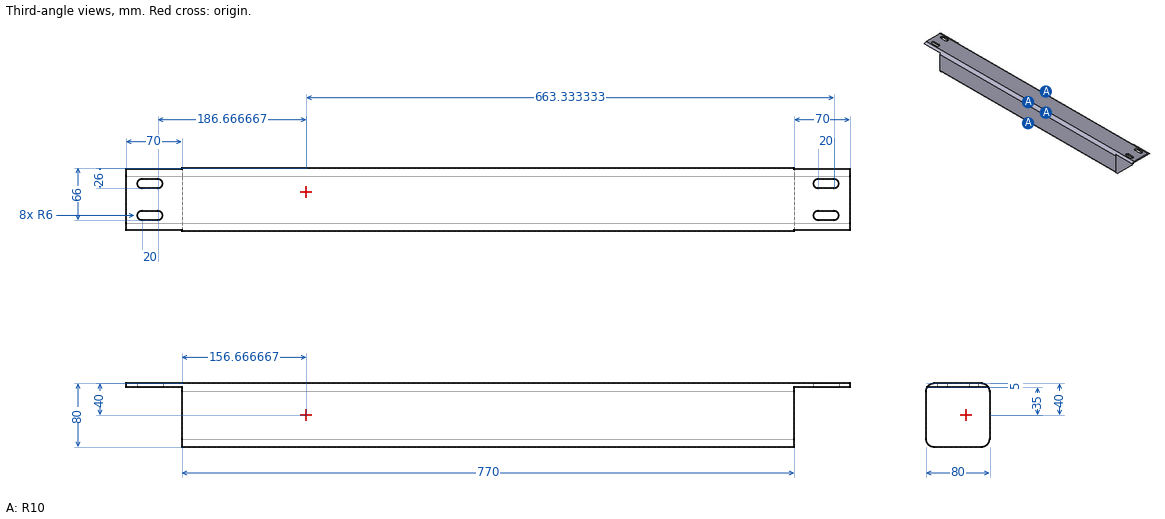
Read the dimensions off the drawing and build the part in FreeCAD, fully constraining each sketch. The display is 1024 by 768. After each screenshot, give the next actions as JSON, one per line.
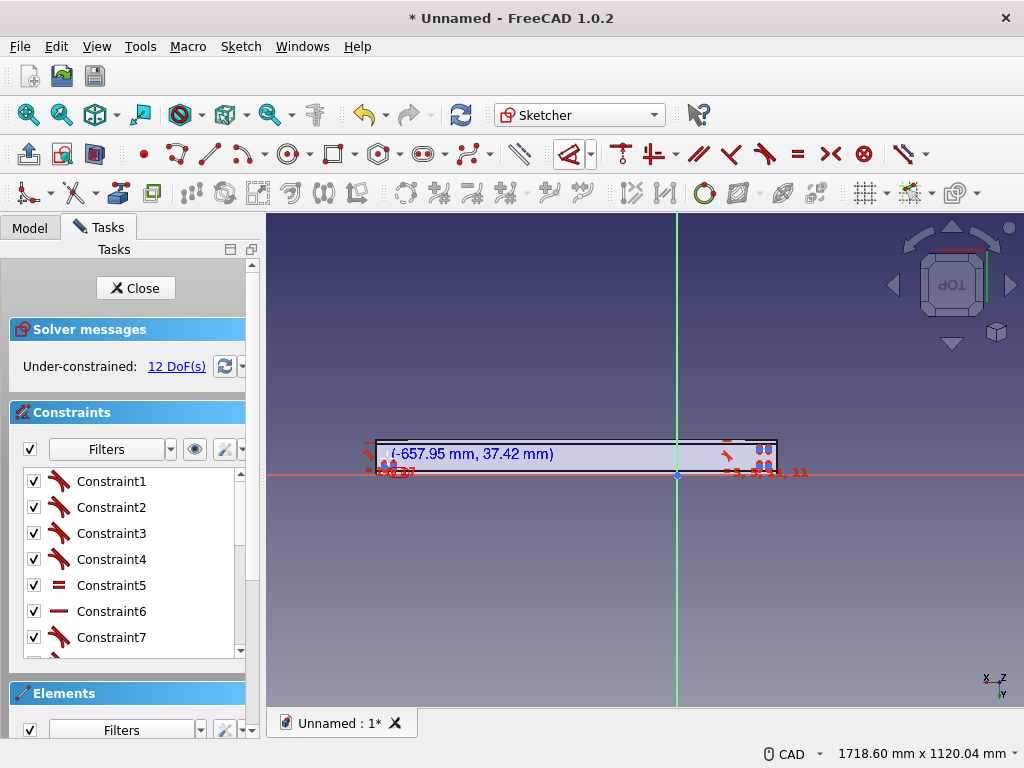
{"action": "left_click", "coordinate": [385, 449]}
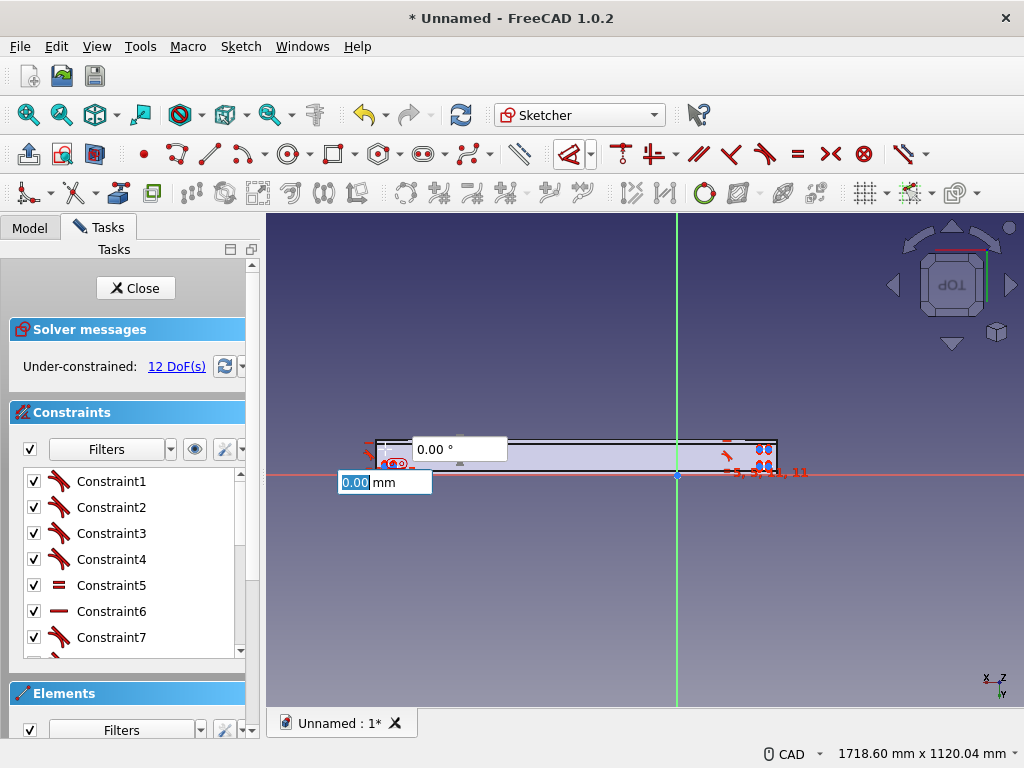
{"action": "scroll", "coordinate": [394, 449], "scroll_direction": "up", "scroll_amount": 3}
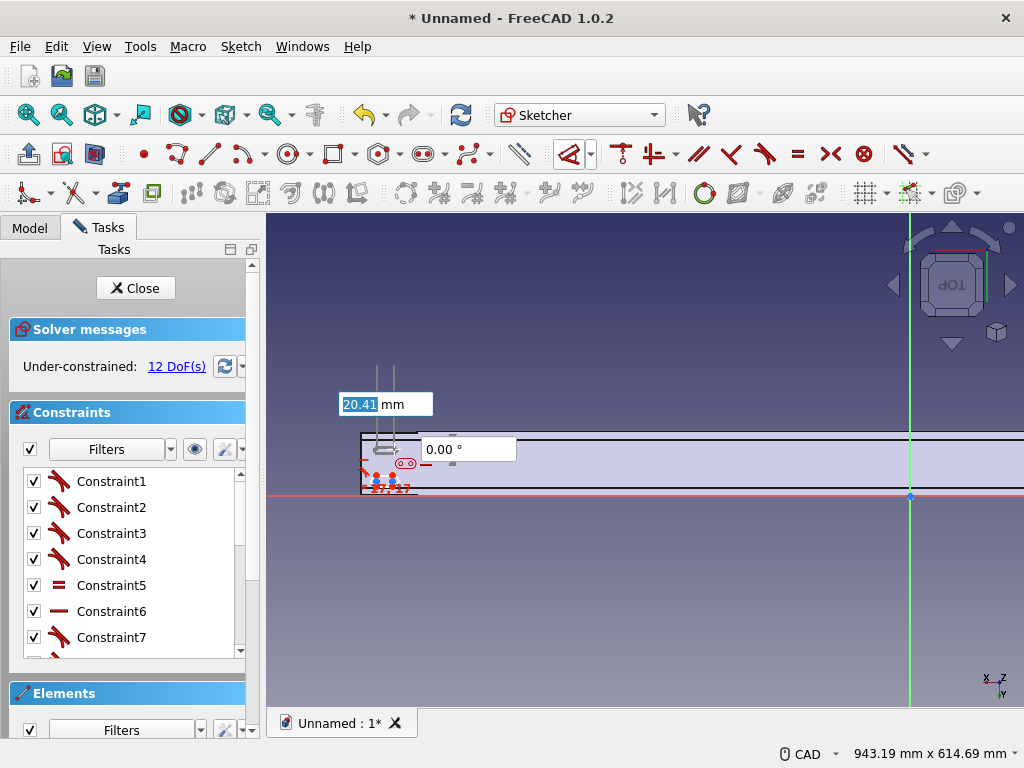
{"action": "left_click", "coordinate": [393, 449]}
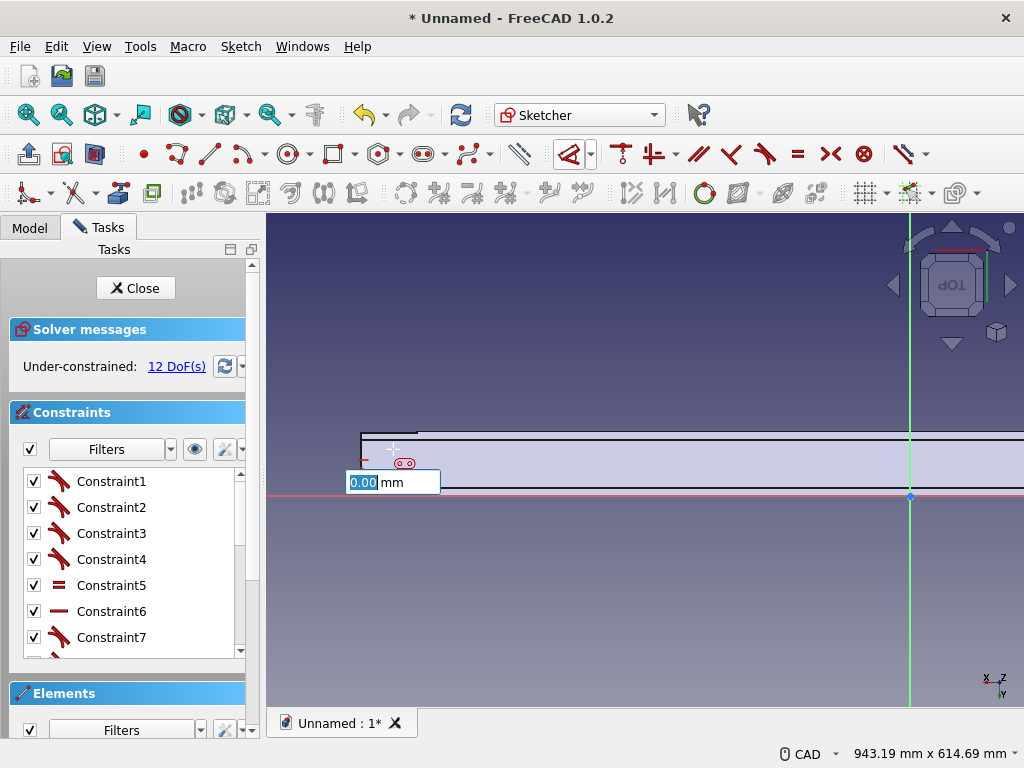
{"action": "scroll", "coordinate": [385, 453], "scroll_direction": "up", "scroll_amount": 6}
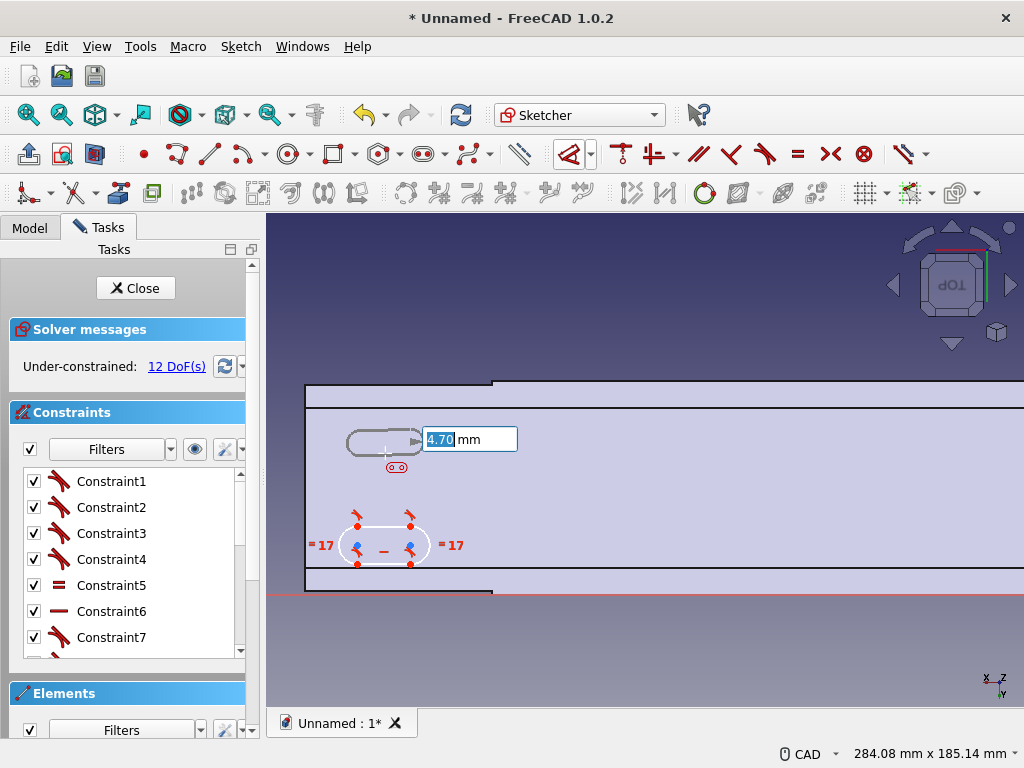
{"action": "left_click", "coordinate": [385, 451]}
{"action": "key", "text": "Escape"}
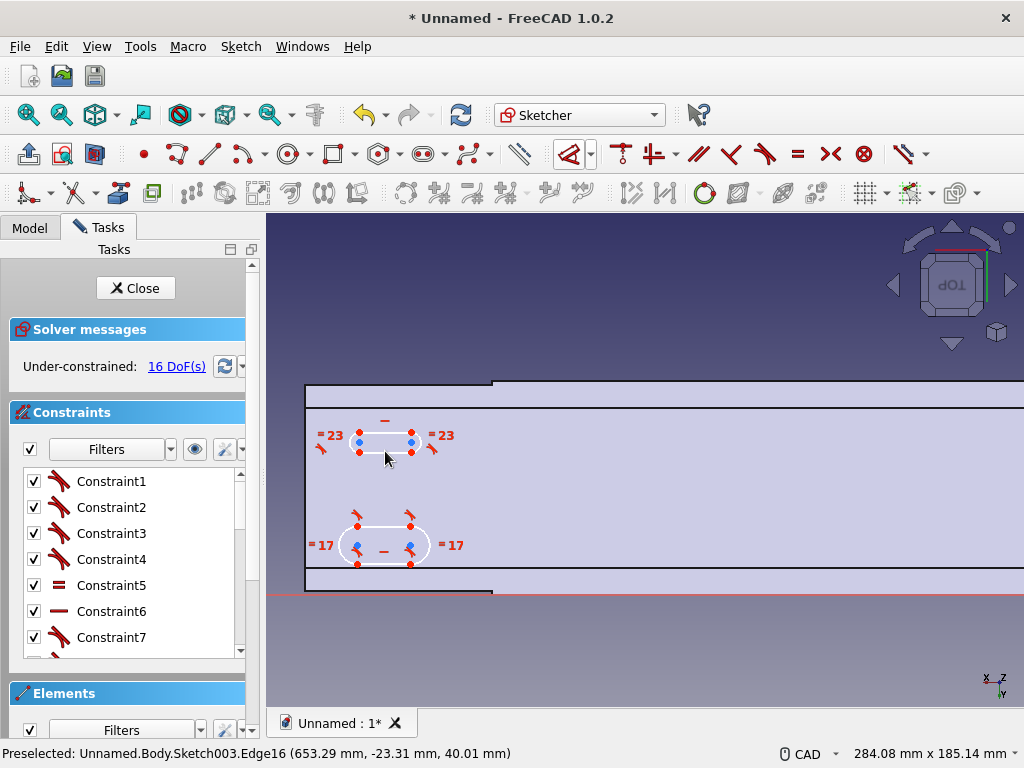
{"action": "scroll", "coordinate": [390, 451], "scroll_direction": "down", "scroll_amount": 9}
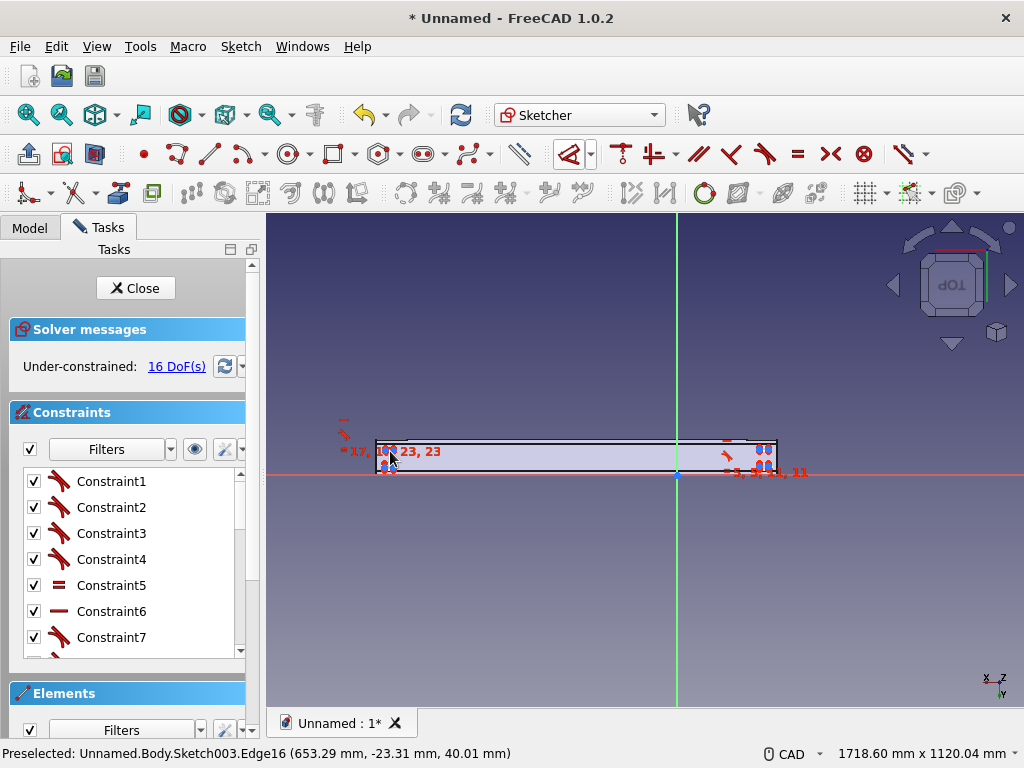
{"action": "scroll", "coordinate": [758, 448], "scroll_direction": "up", "scroll_amount": 11}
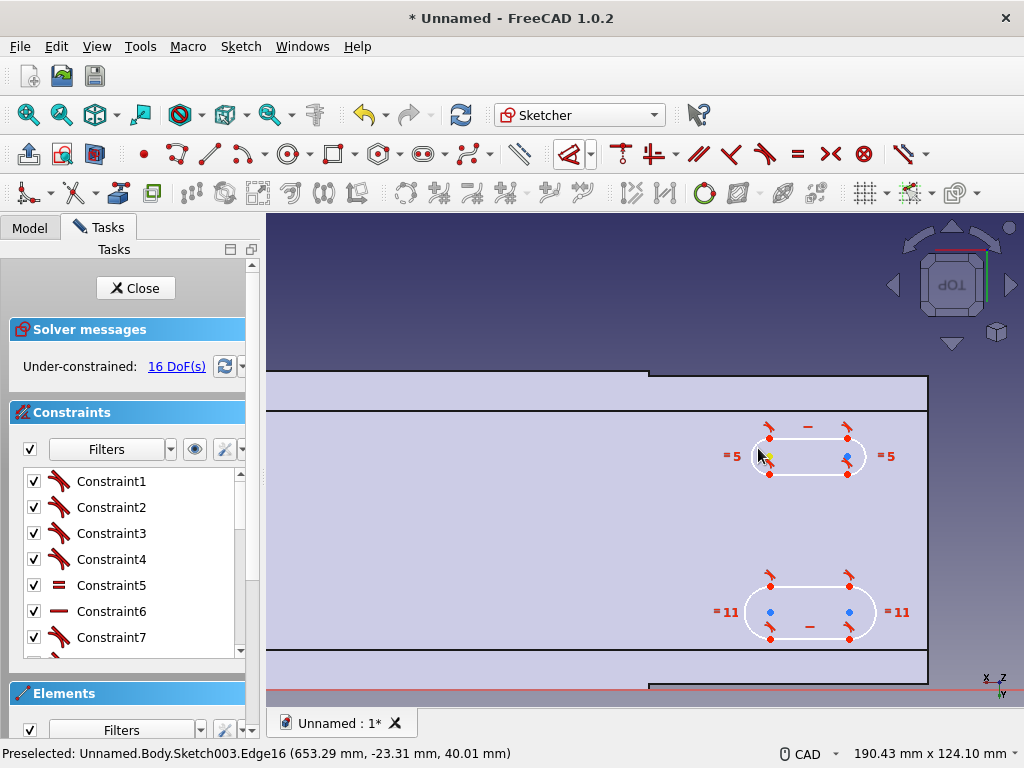
{"action": "left_click", "coordinate": [755, 446]}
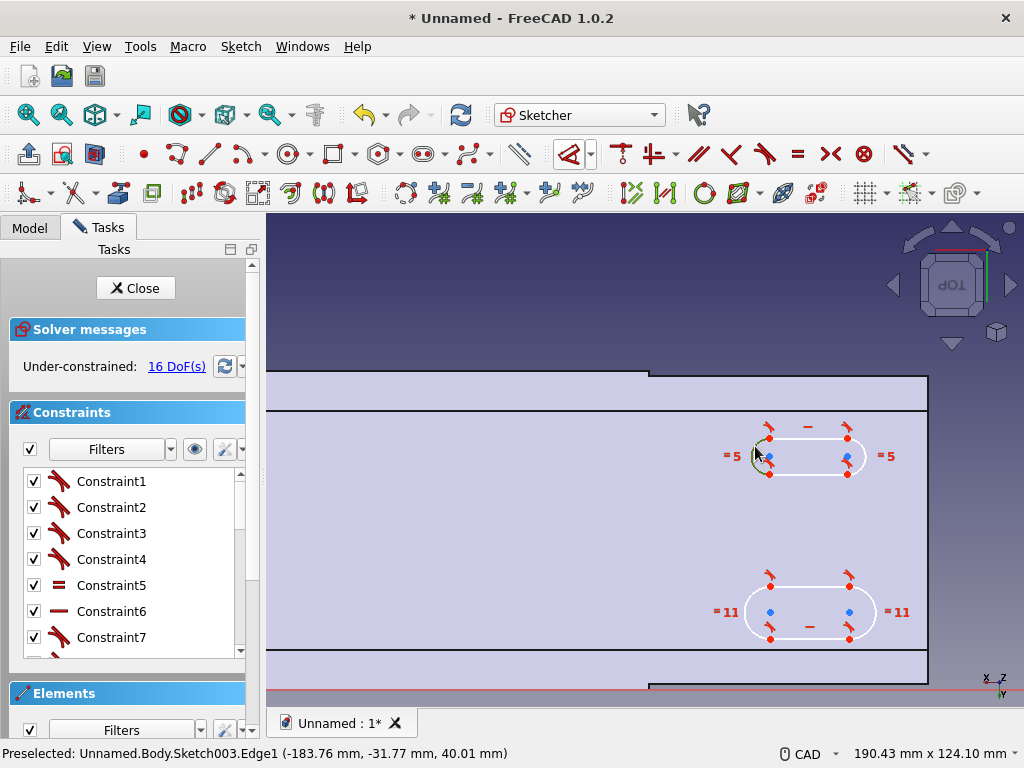
{"action": "left_click", "coordinate": [750, 598]}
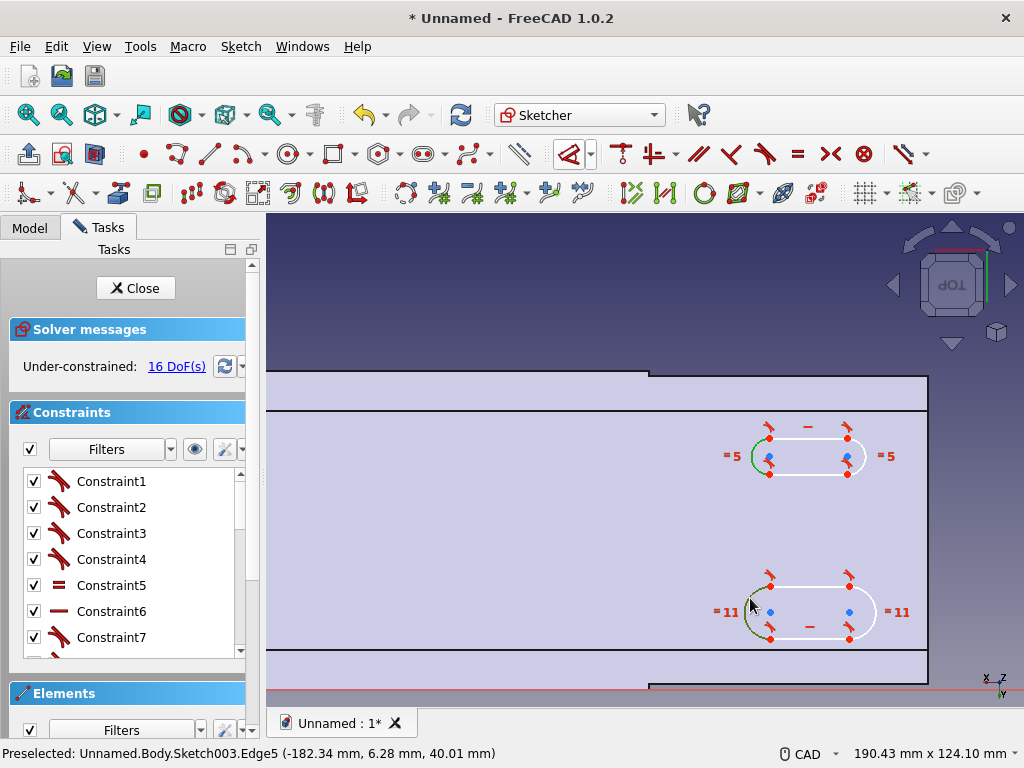
{"action": "scroll", "coordinate": [758, 448], "scroll_direction": "down", "scroll_amount": 11}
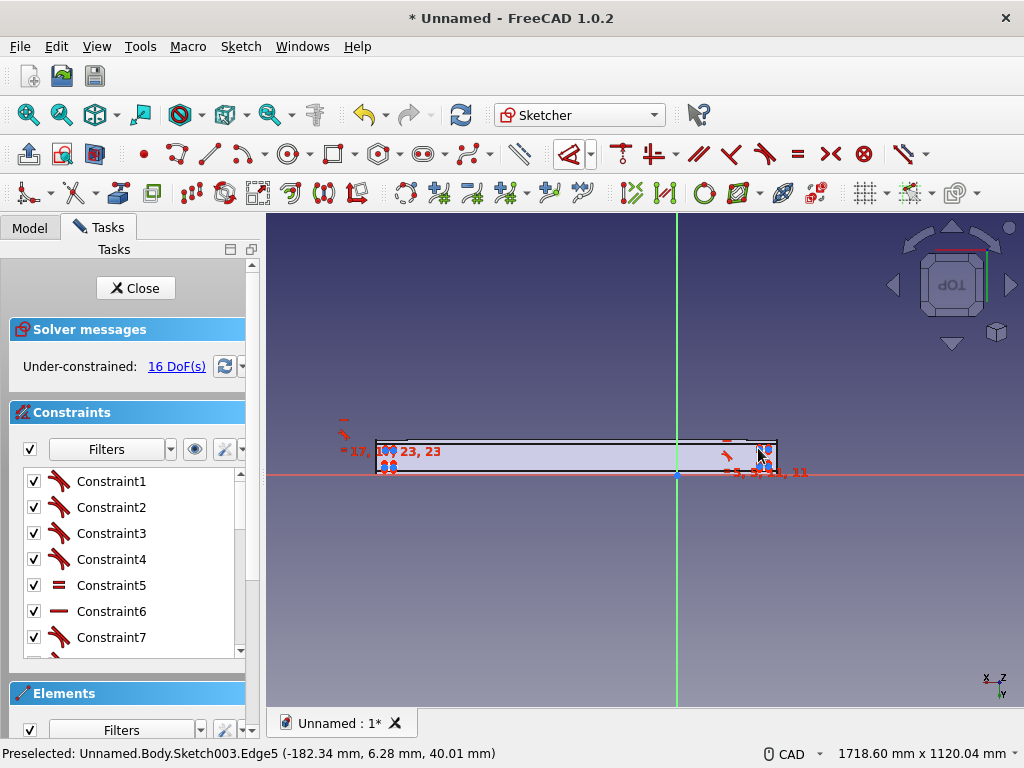
{"action": "scroll", "coordinate": [382, 465], "scroll_direction": "up", "scroll_amount": 8}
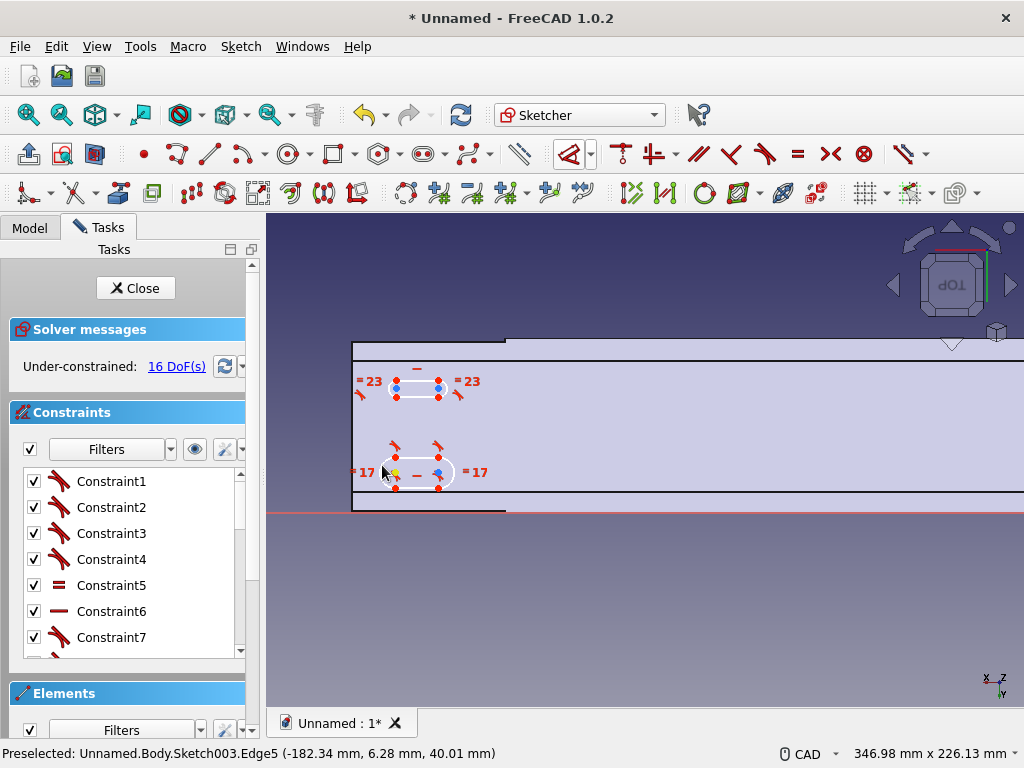
{"action": "left_click", "coordinate": [383, 464]}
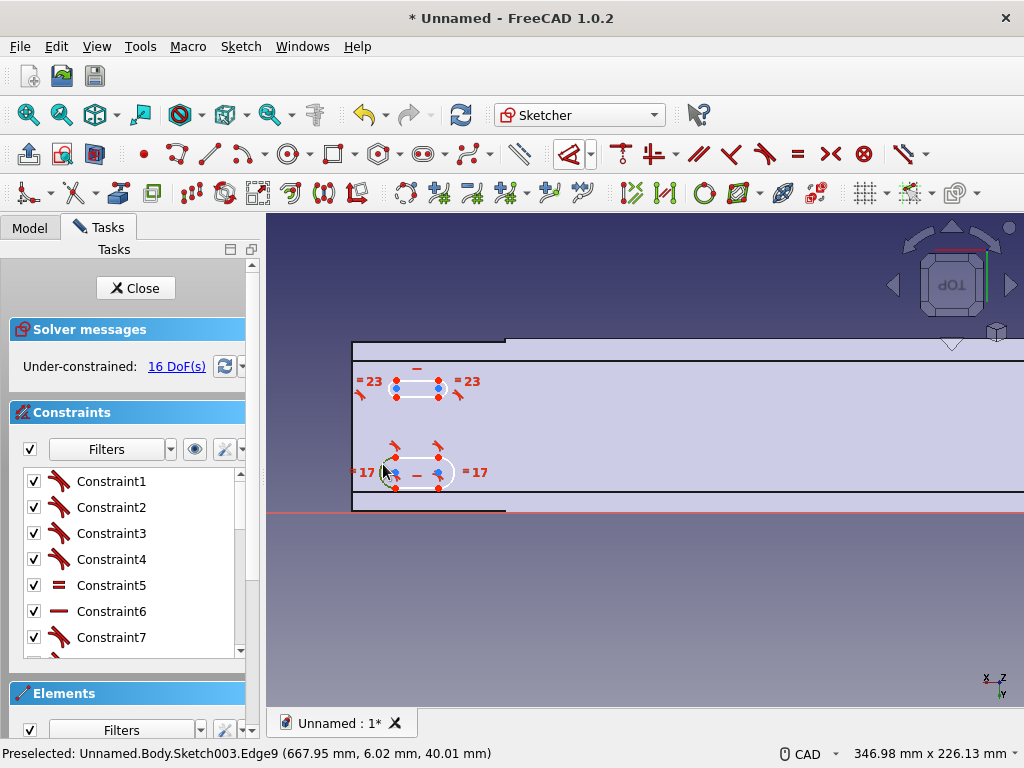
{"action": "scroll", "coordinate": [389, 389], "scroll_direction": "up", "scroll_amount": 3}